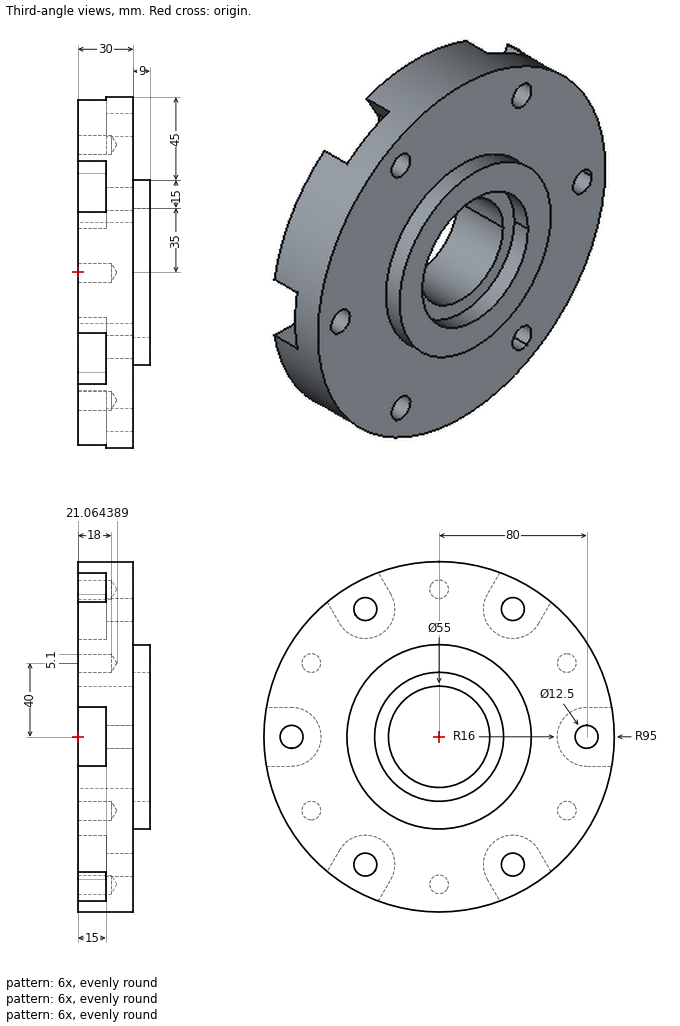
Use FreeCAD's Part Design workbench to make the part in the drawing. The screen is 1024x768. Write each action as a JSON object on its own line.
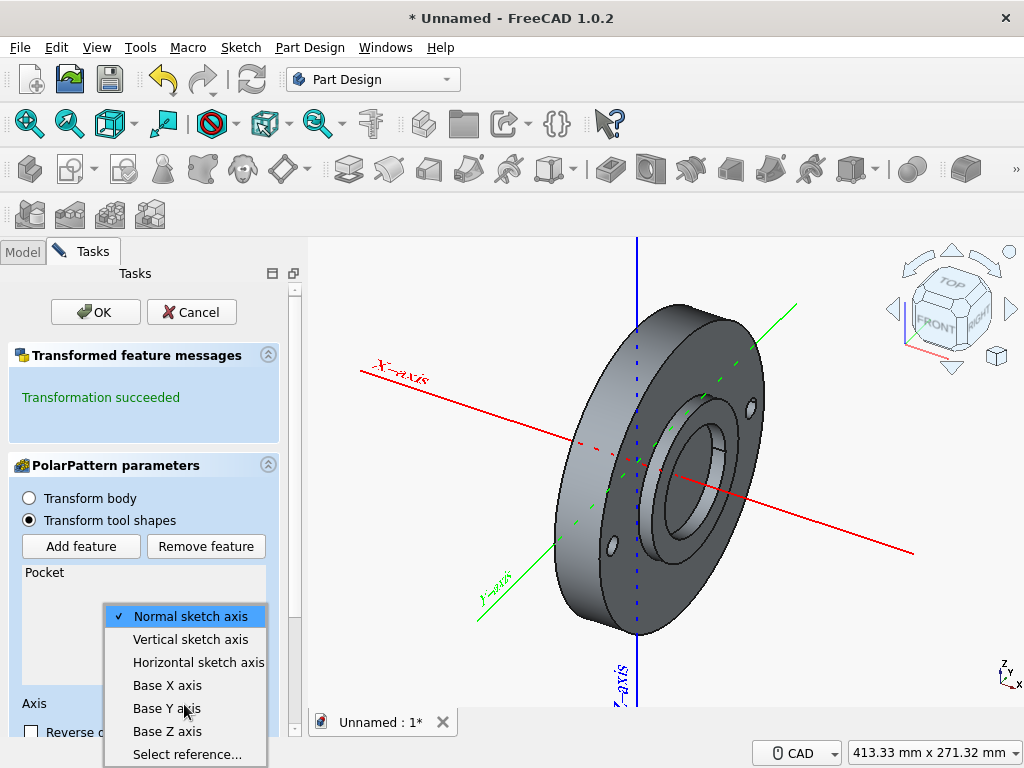
{"action": "left_click", "coordinate": [184, 686]}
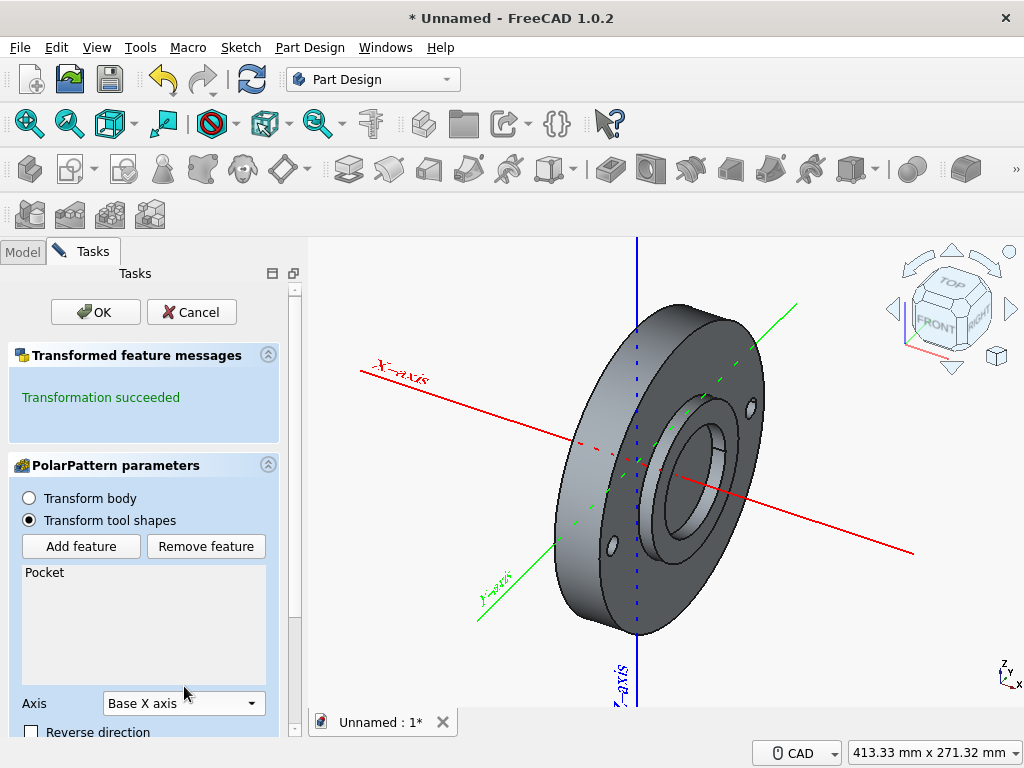
{"action": "scroll", "coordinate": [295, 510], "scroll_direction": "down", "scroll_amount": 3}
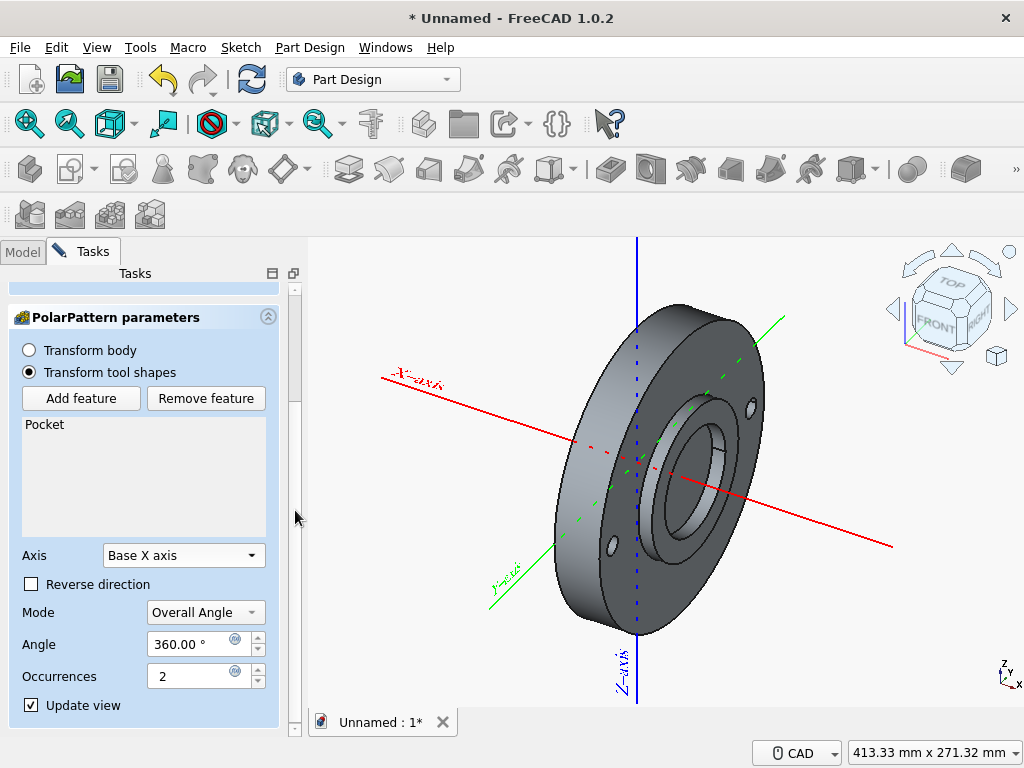
{"action": "triple_click", "coordinate": [198, 676]}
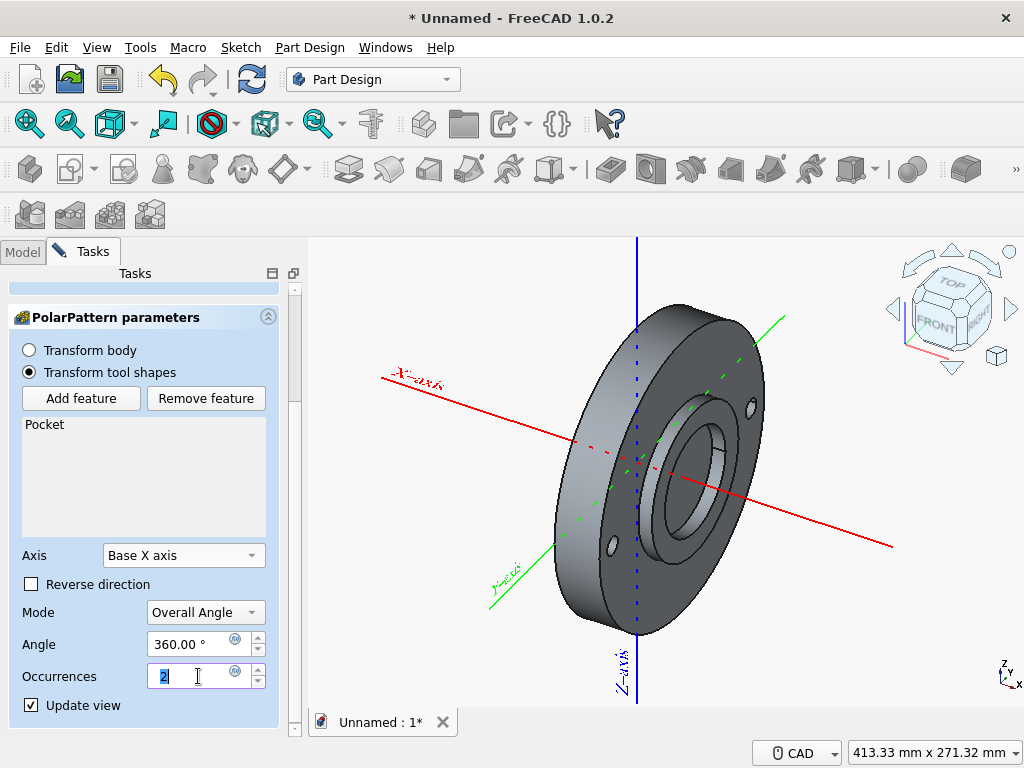
{"action": "type", "text": "6"}
{"action": "key", "text": "Tab"}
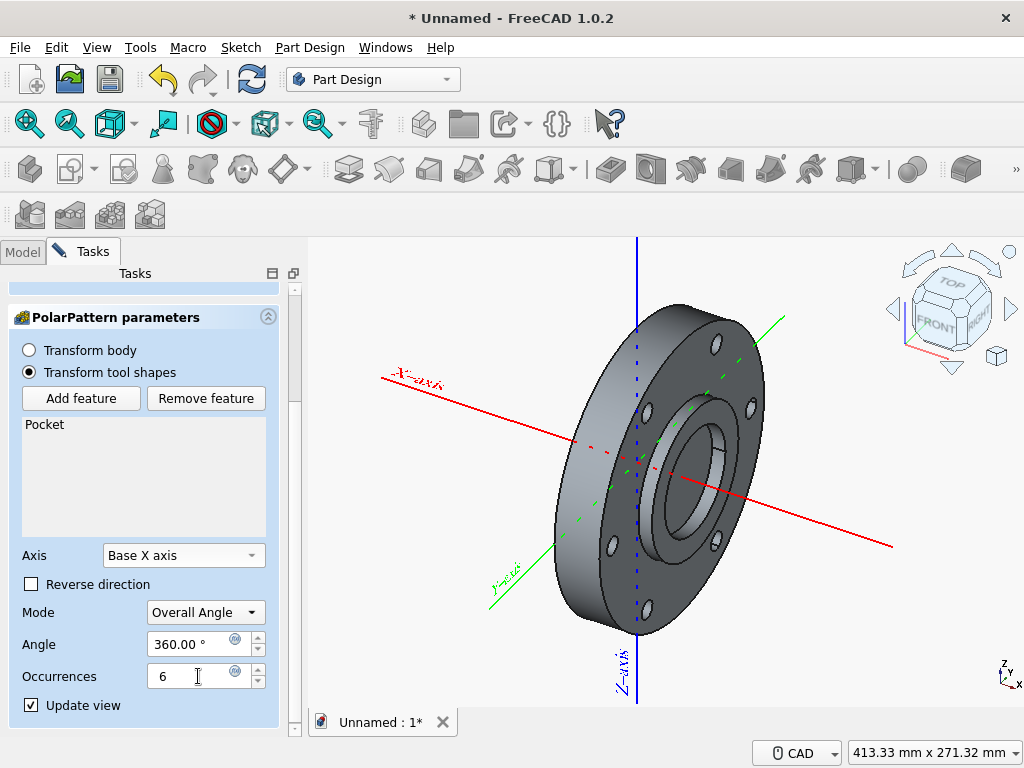
{"action": "scroll", "coordinate": [295, 510], "scroll_direction": "up", "scroll_amount": 4}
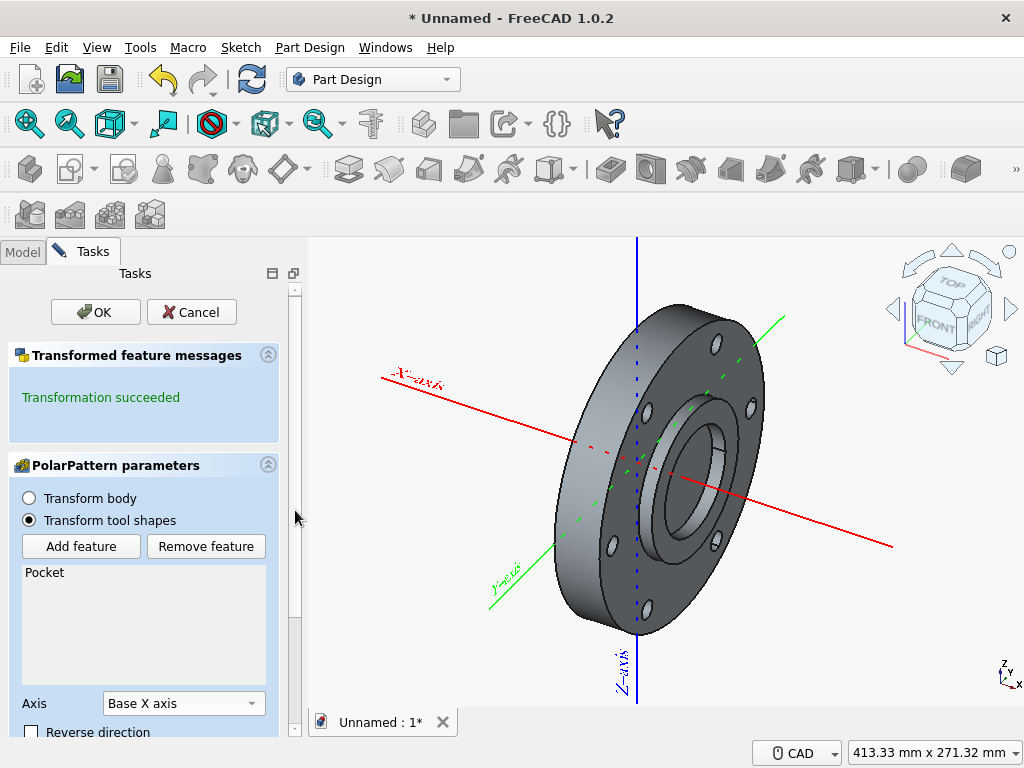
{"action": "left_click", "coordinate": [96, 312]}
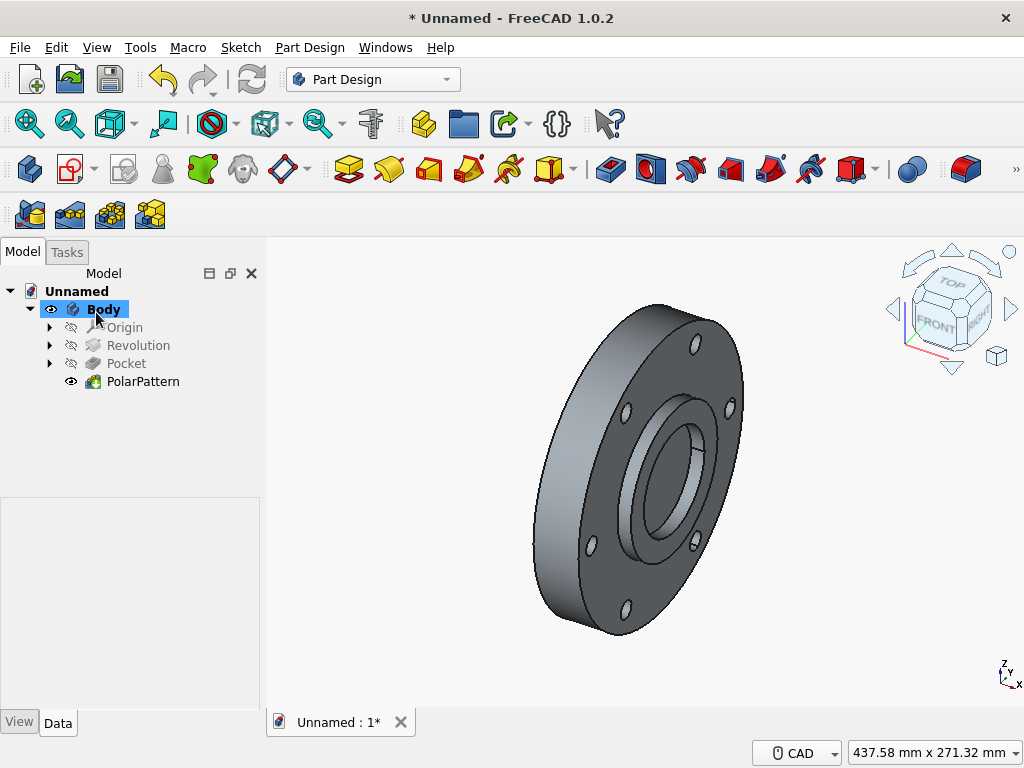
{"action": "left_click", "coordinate": [70, 170]}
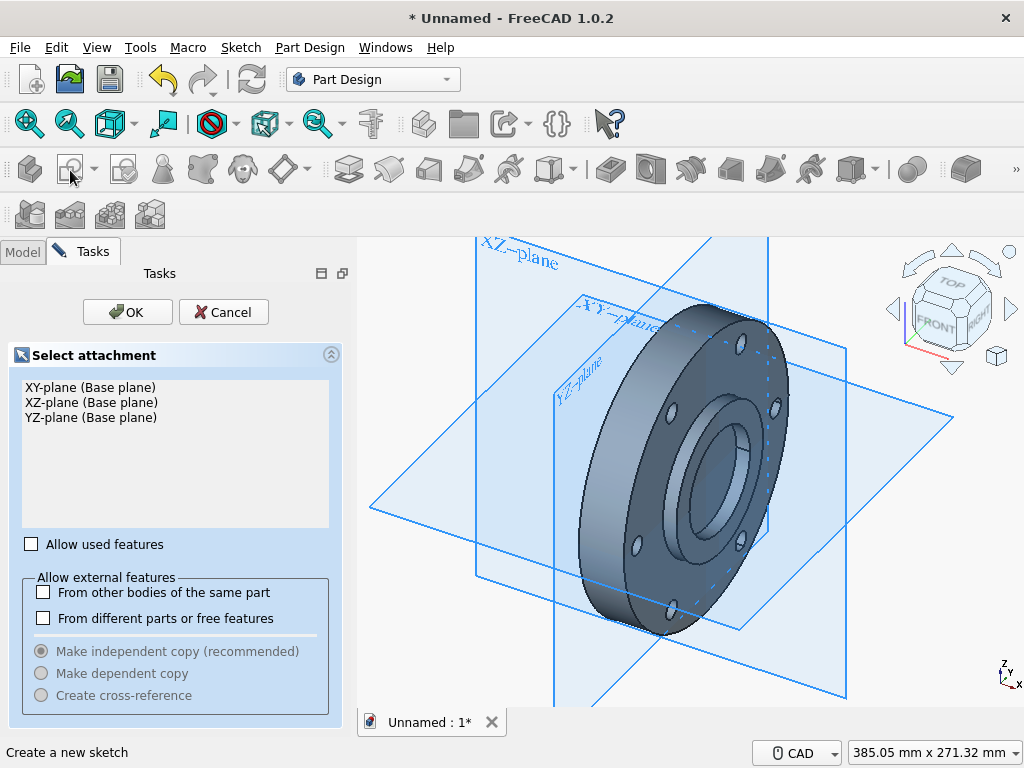
{"action": "left_click", "coordinate": [82, 418]}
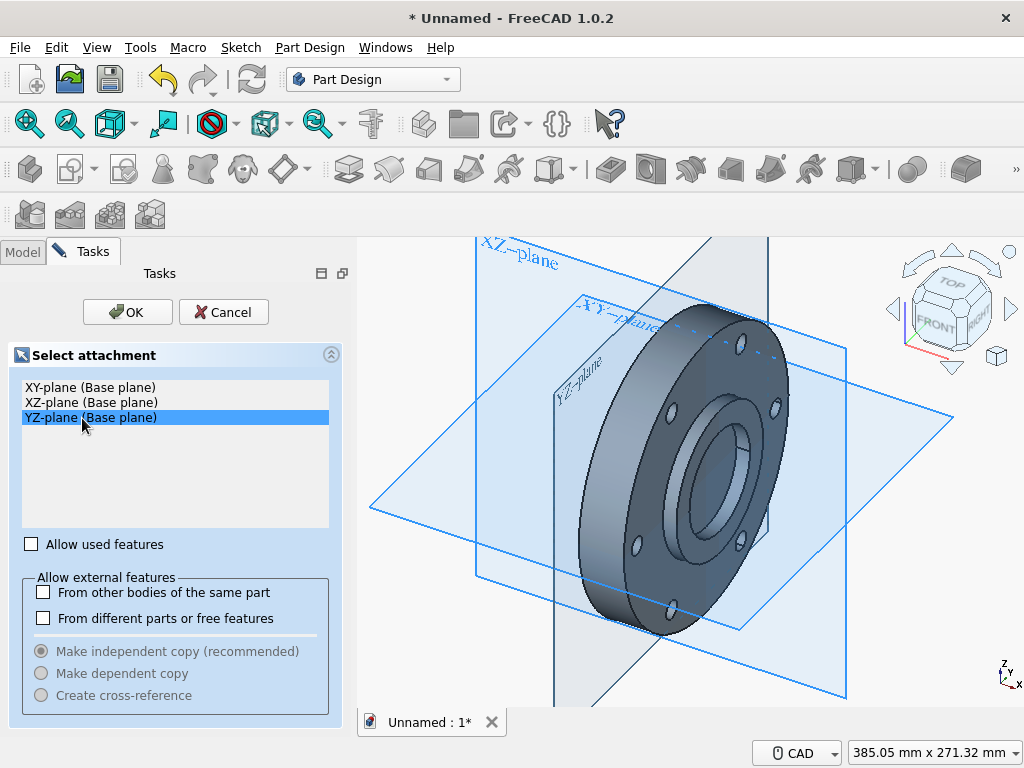
{"action": "left_click", "coordinate": [128, 312]}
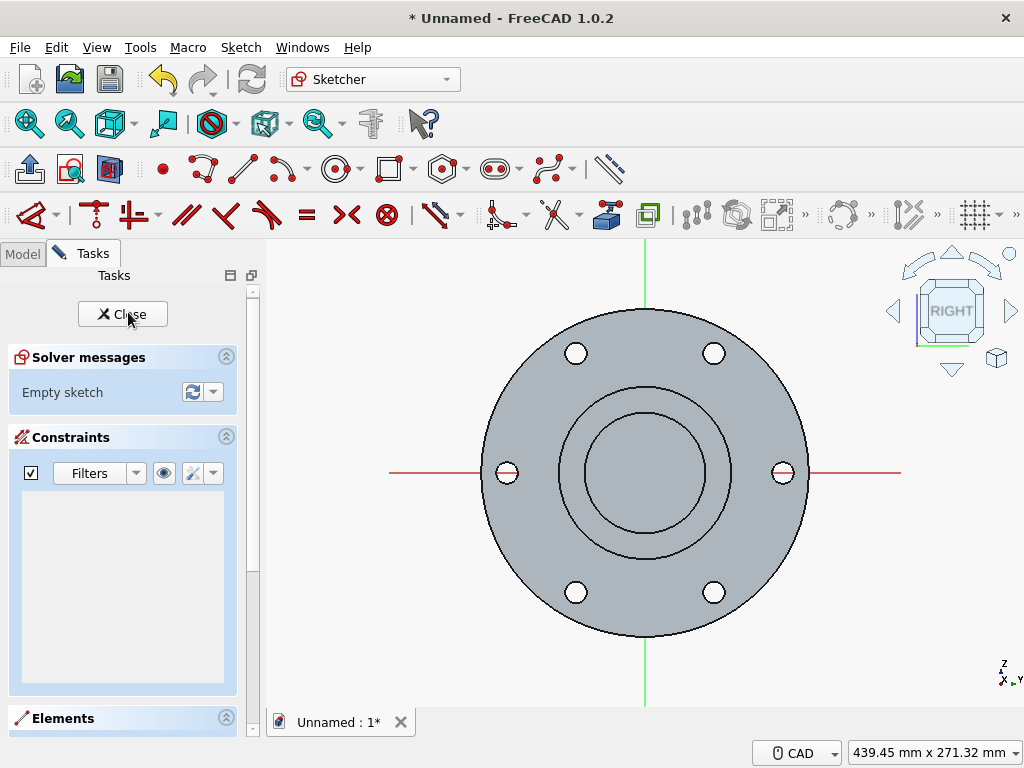
{"action": "left_click", "coordinate": [110, 170]}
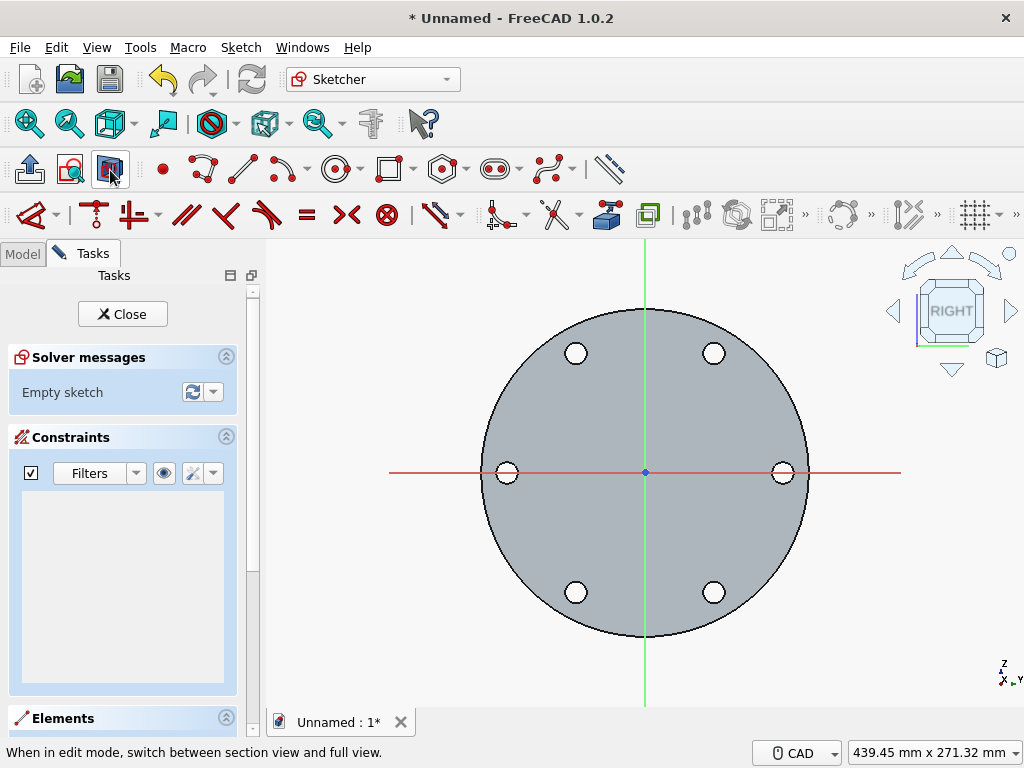
{"action": "scroll", "coordinate": [675, 473], "scroll_direction": "up", "scroll_amount": 6}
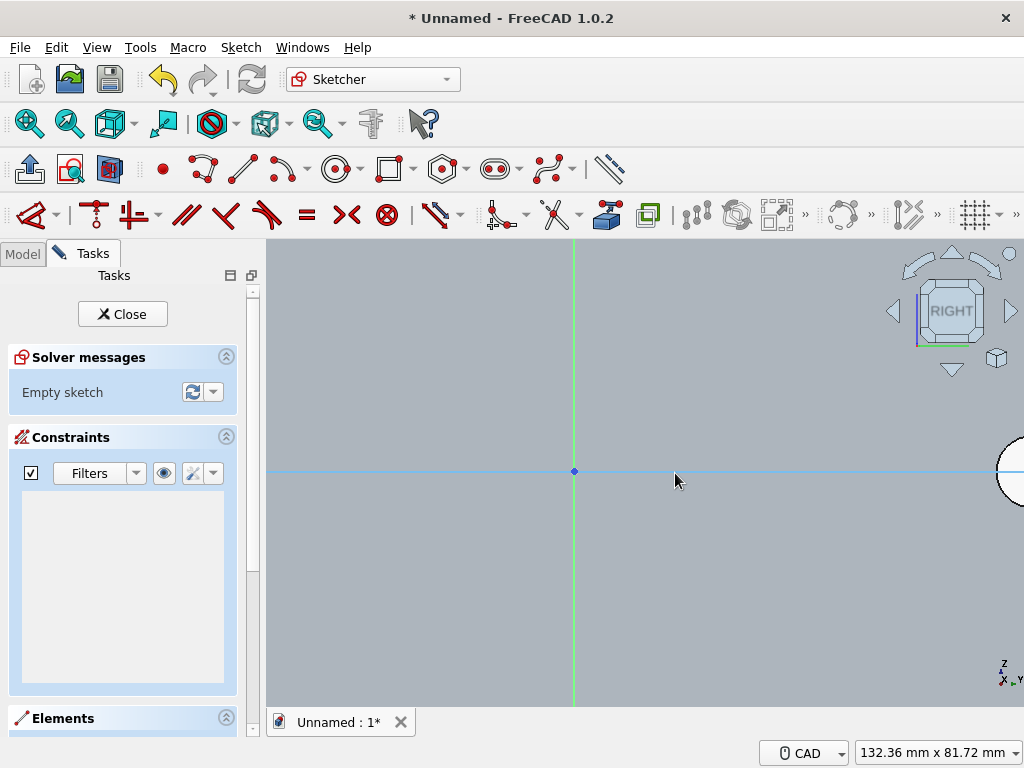
{"action": "left_click", "coordinate": [336, 170]}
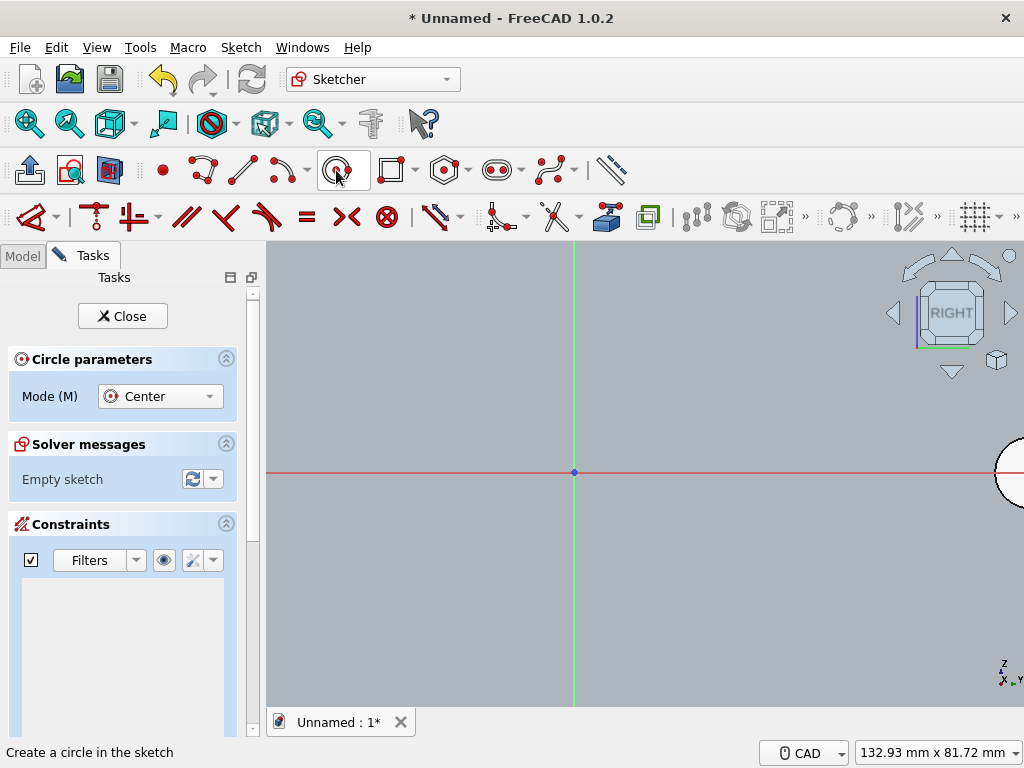
{"action": "left_click", "coordinate": [574, 473]}
{"action": "mouse_move", "coordinate": [685, 362]}